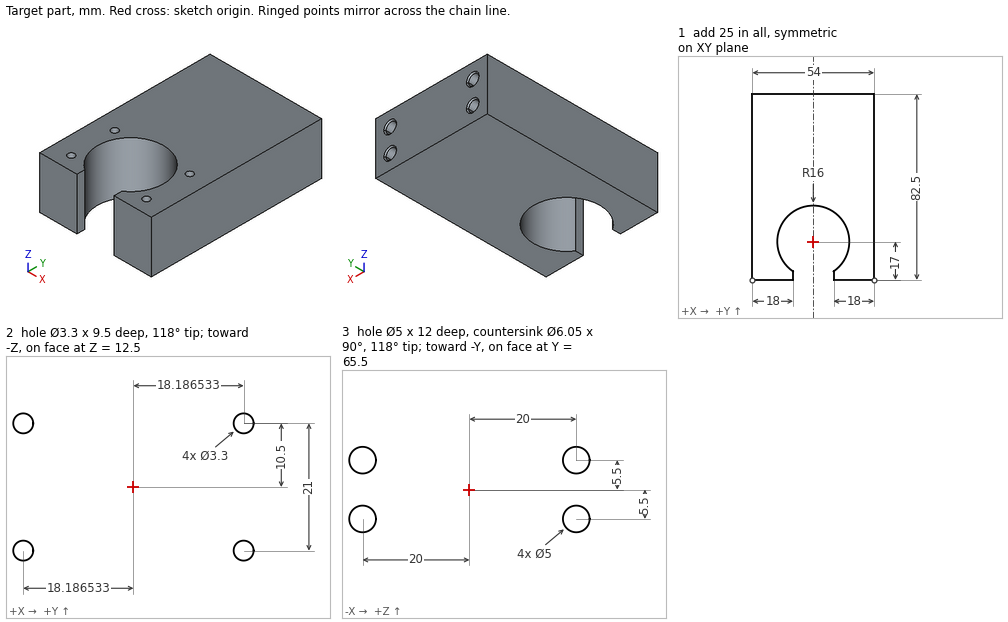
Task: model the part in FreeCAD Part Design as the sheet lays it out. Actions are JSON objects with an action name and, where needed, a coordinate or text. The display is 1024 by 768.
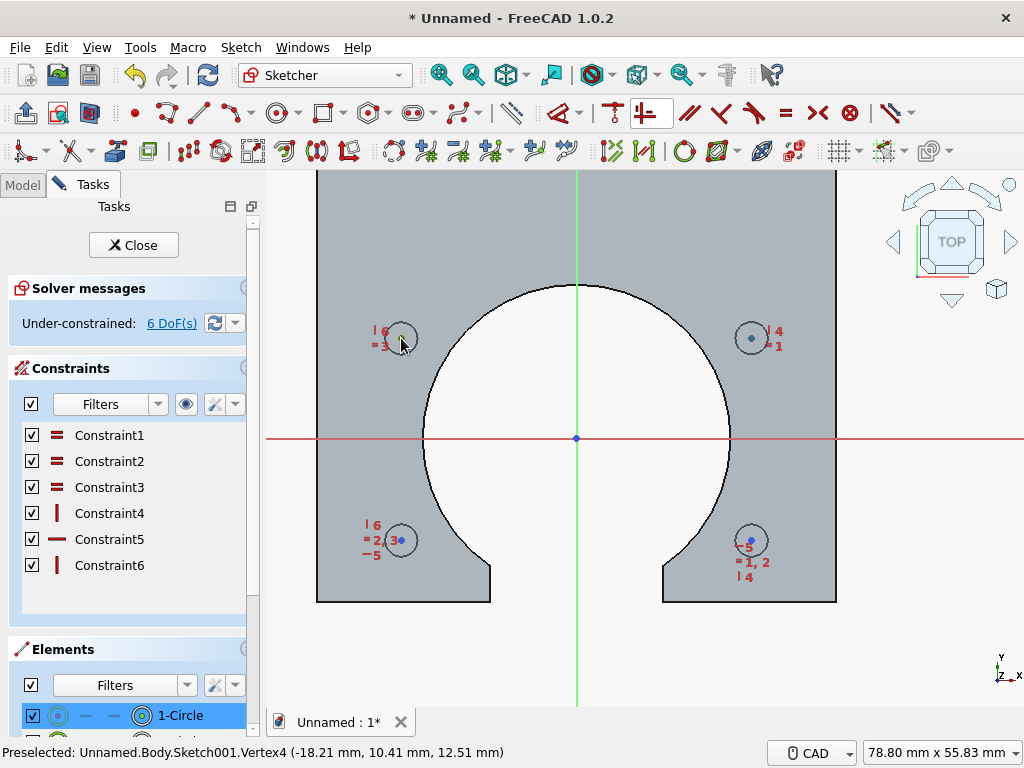
{"action": "key", "text": "h"}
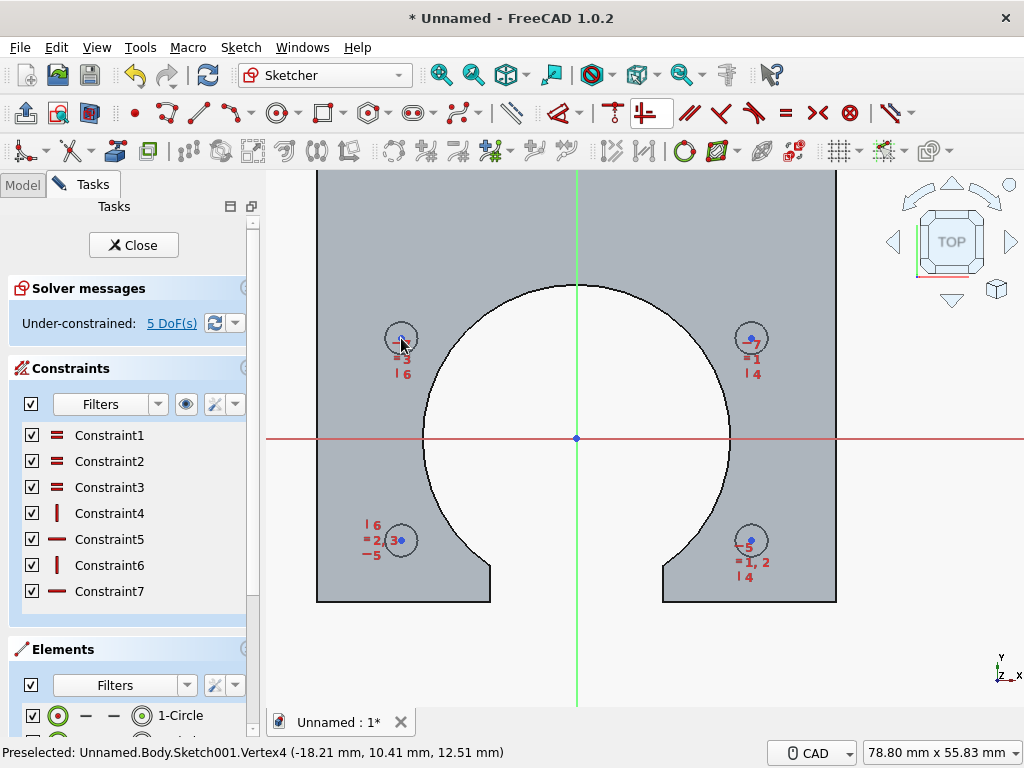
{"action": "left_click", "coordinate": [558, 114]}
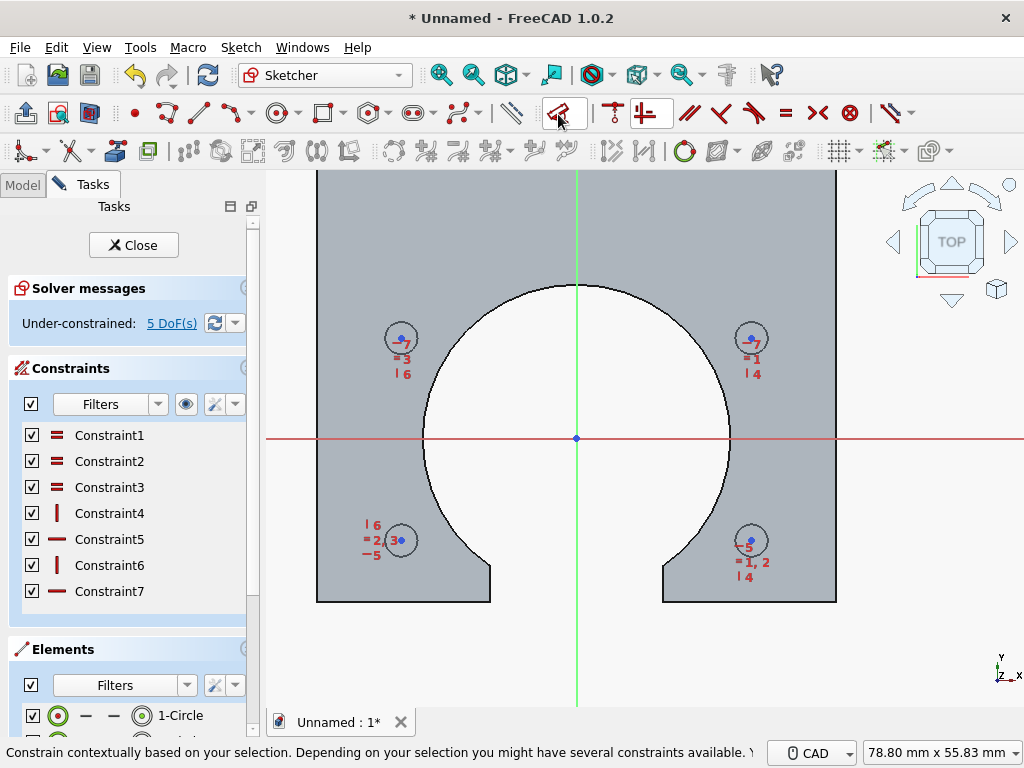
{"action": "scroll", "coordinate": [763, 327], "scroll_direction": "up", "scroll_amount": 2}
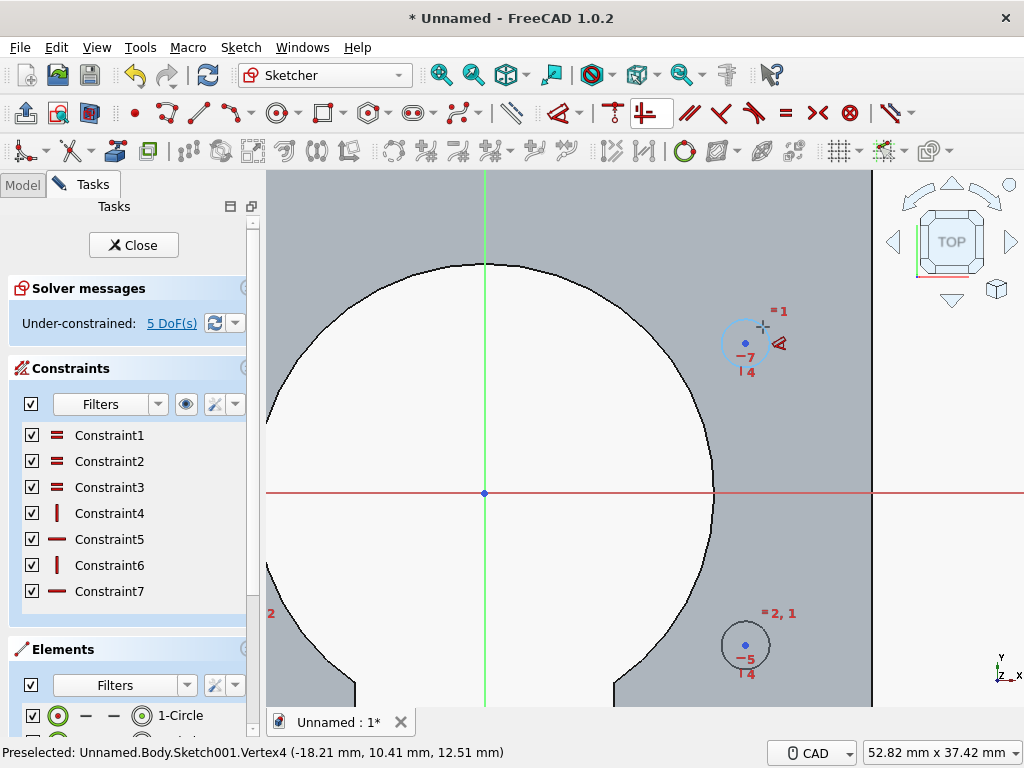
{"action": "left_click", "coordinate": [763, 326]}
{"action": "left_click", "coordinate": [786, 303]}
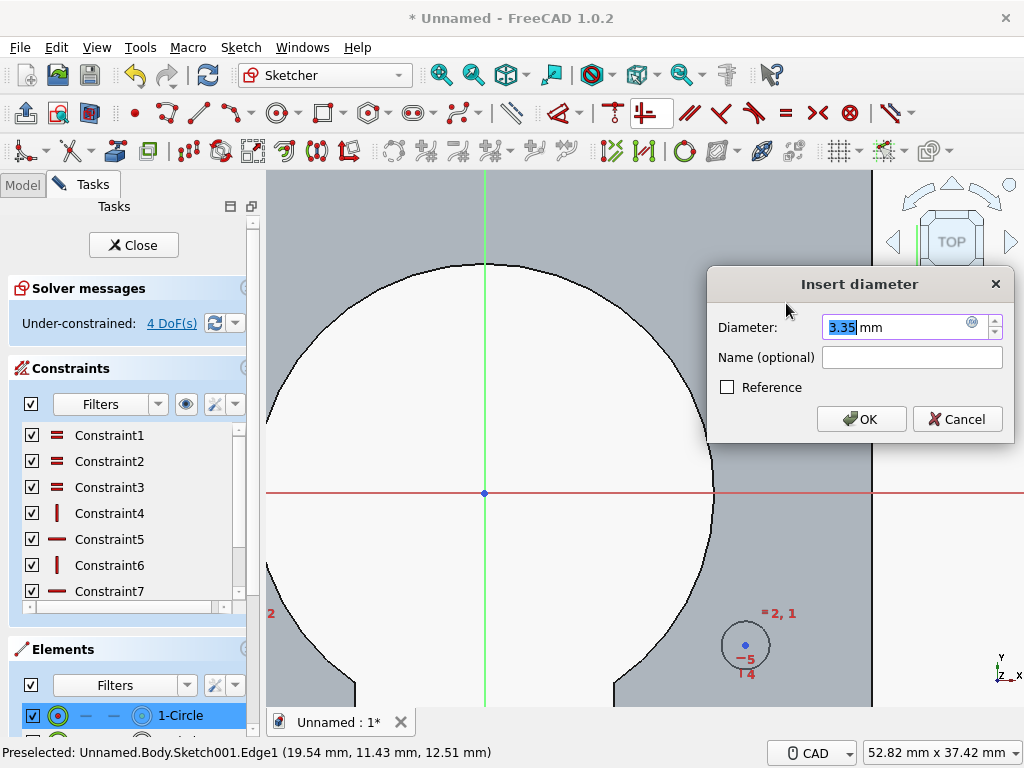
{"action": "type", "text": "3.3"}
{"action": "key", "text": "Return"}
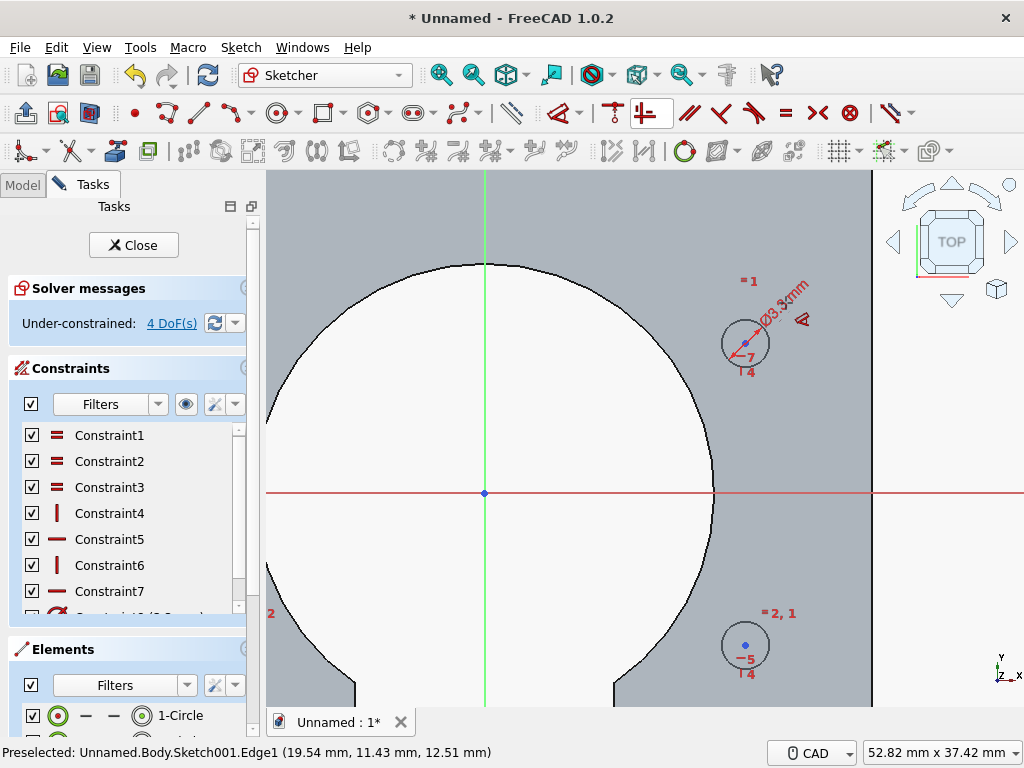
{"action": "left_click", "coordinate": [746, 343]}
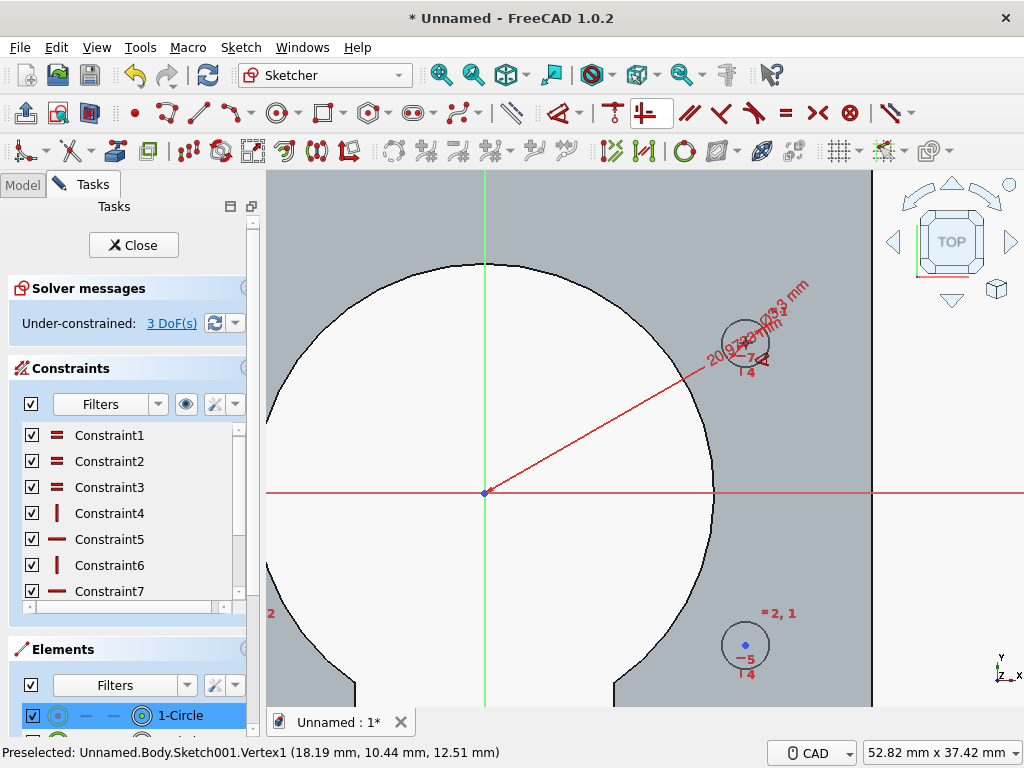
{"action": "left_click", "coordinate": [746, 645]}
{"action": "left_click", "coordinate": [780, 425]}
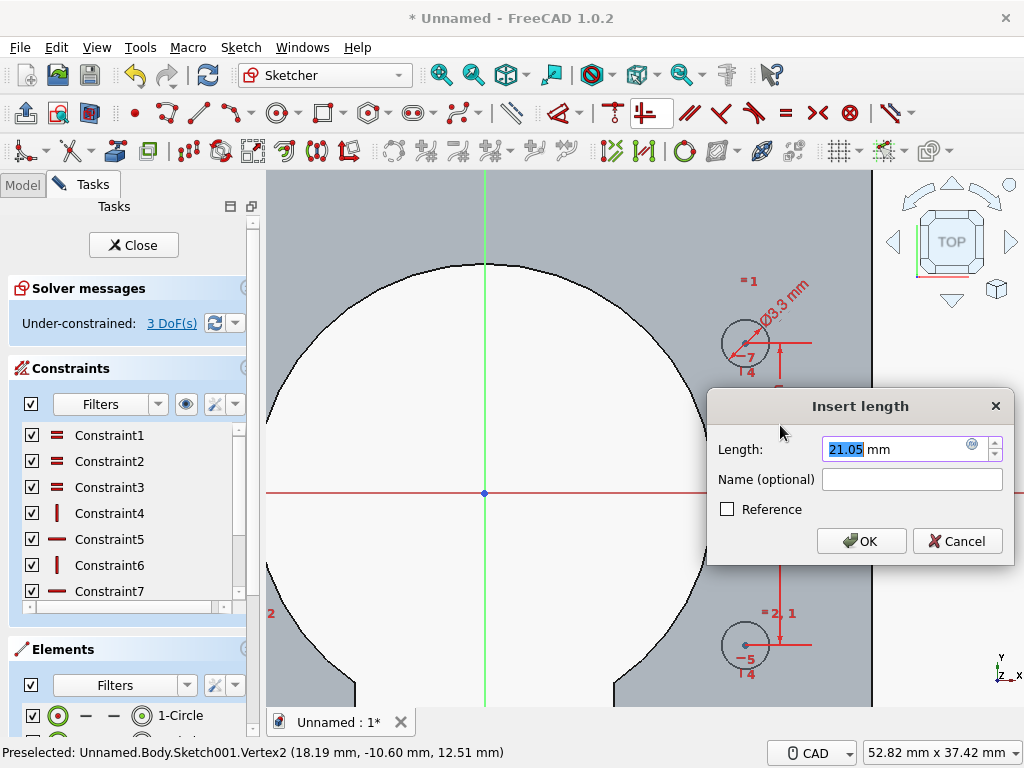
{"action": "type", "text": "21"}
{"action": "key", "text": "Return"}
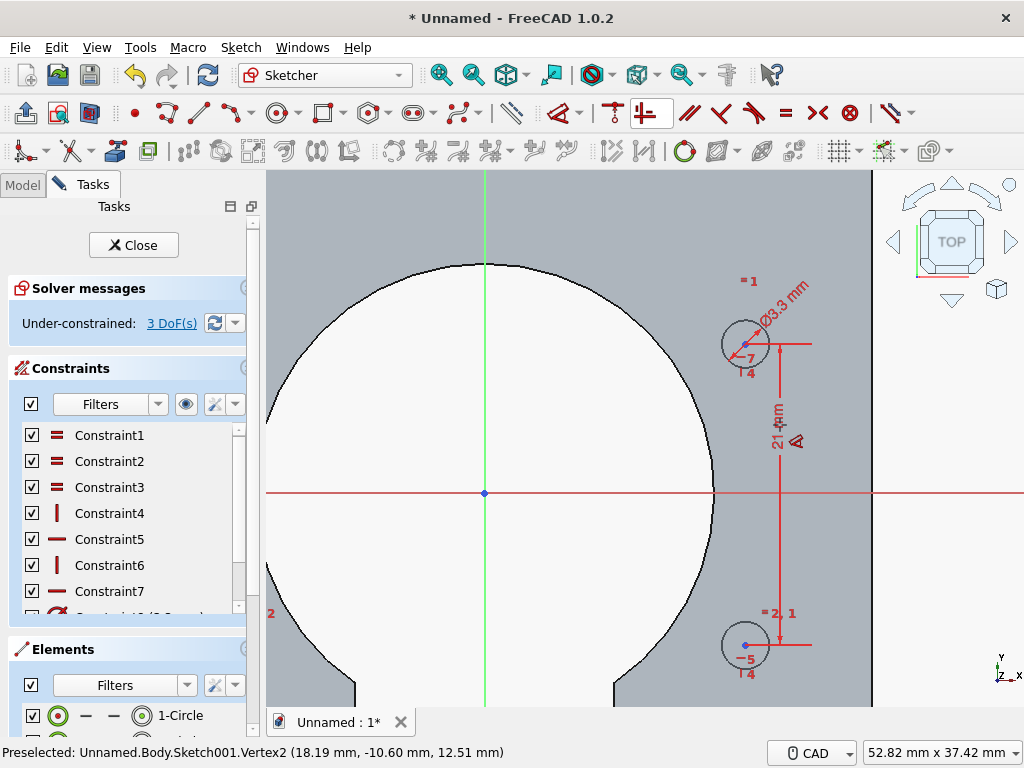
{"action": "left_click", "coordinate": [746, 344]}
{"action": "left_click", "coordinate": [780, 384]}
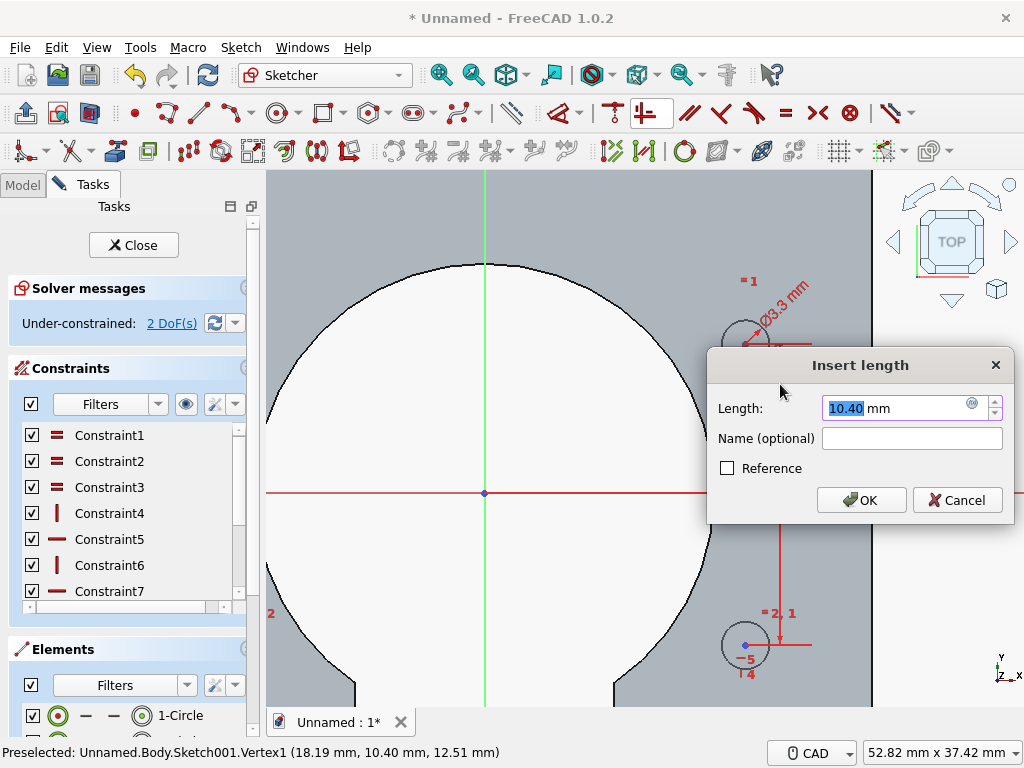
{"action": "type", "text": "10.5"}
{"action": "key", "text": "Return"}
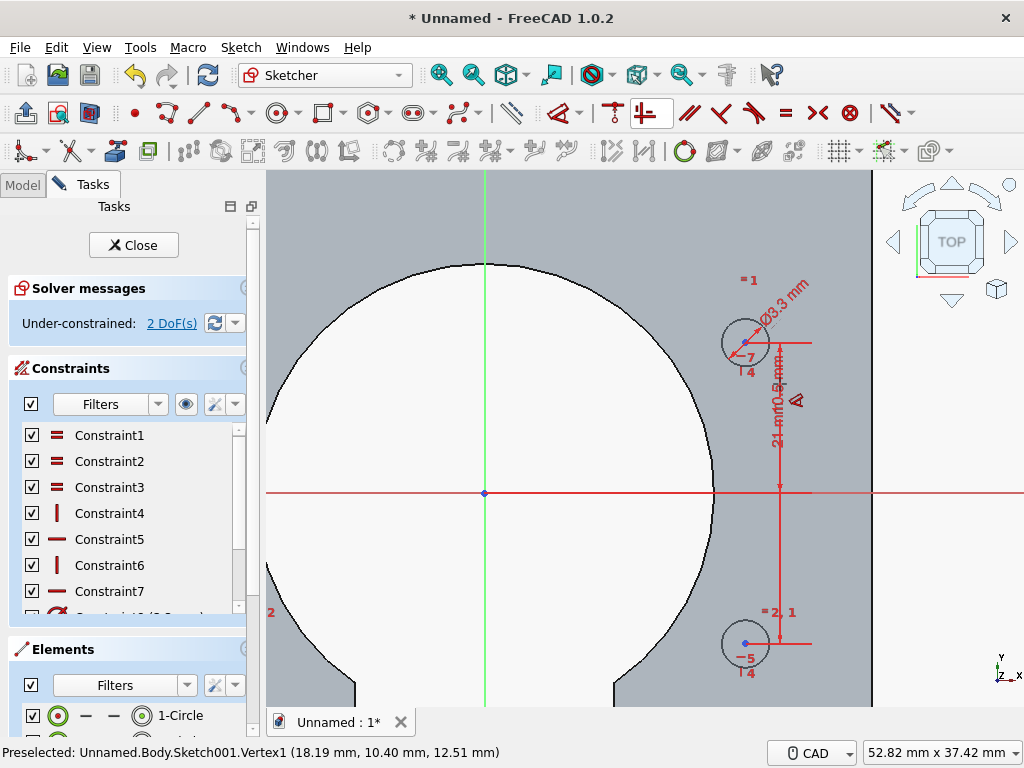
{"action": "left_click", "coordinate": [746, 343]}
{"action": "left_click", "coordinate": [615, 309]}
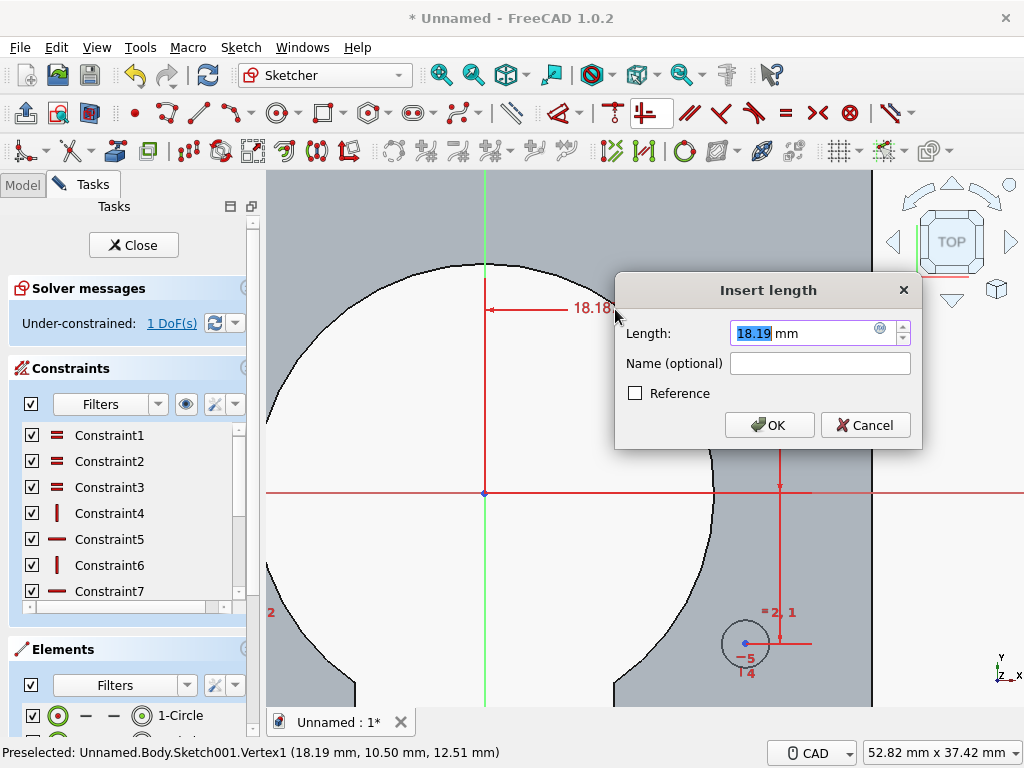
{"action": "type", "text": "18.186533"}
{"action": "key", "text": "Return"}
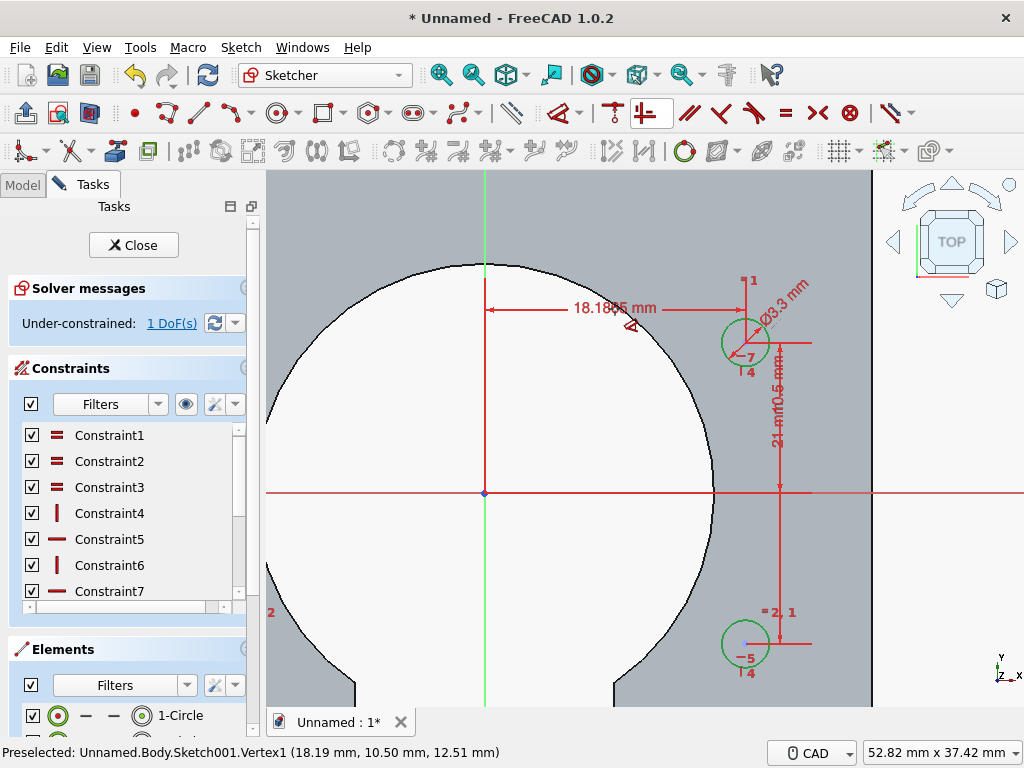
{"action": "scroll", "coordinate": [763, 327], "scroll_direction": "down", "scroll_amount": 2}